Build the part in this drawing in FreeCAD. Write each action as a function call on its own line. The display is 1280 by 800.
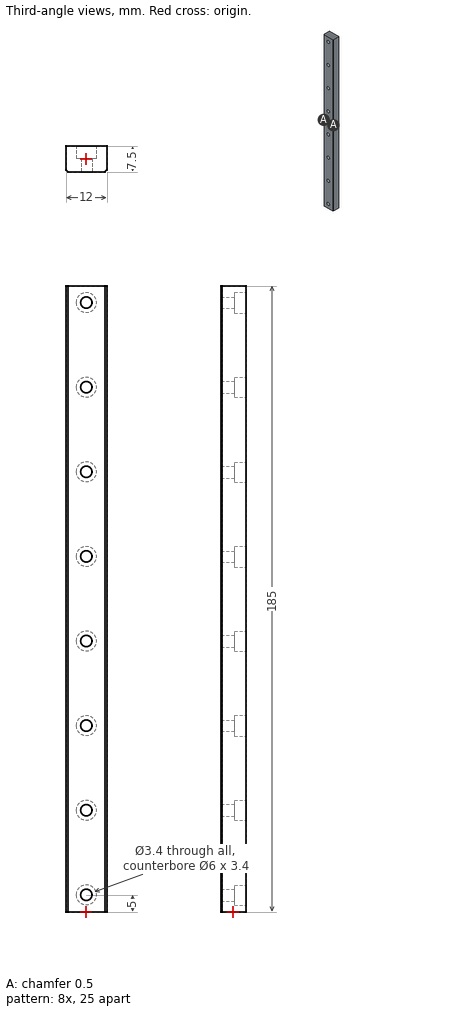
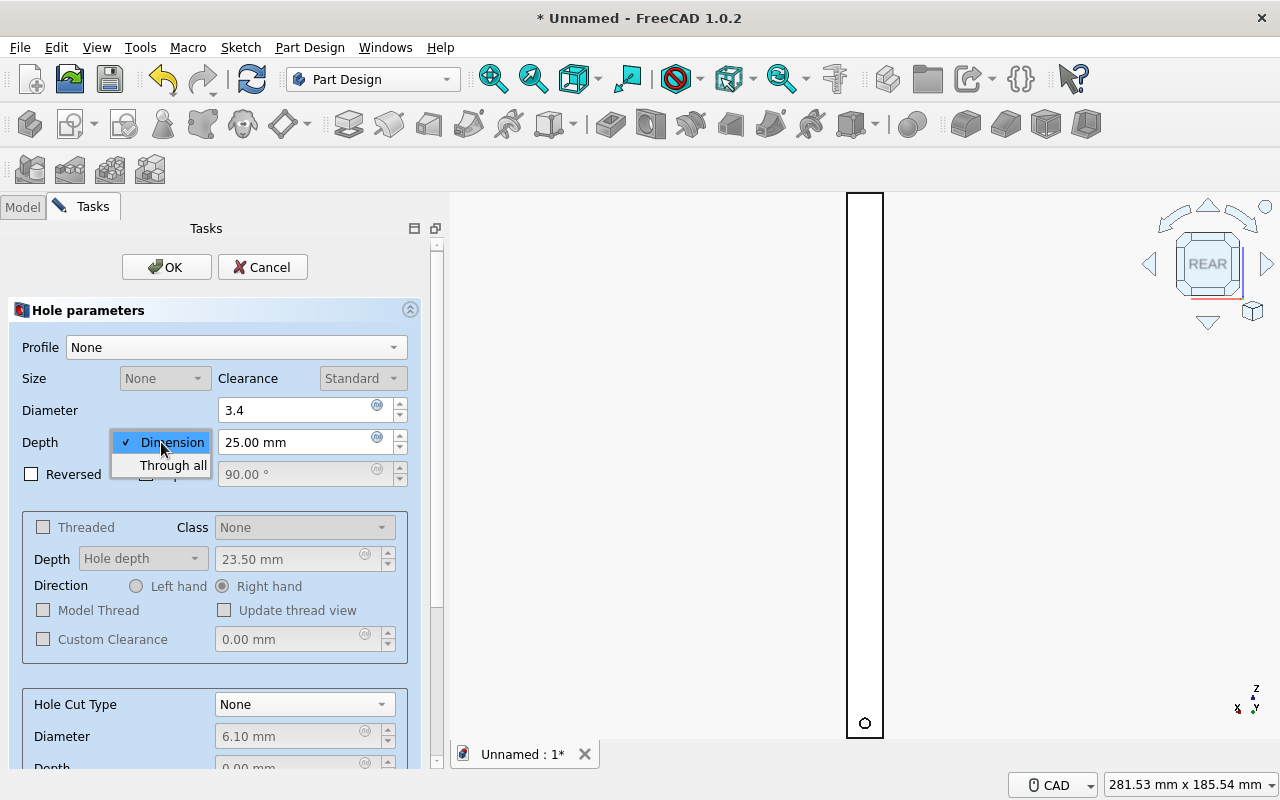
click(160, 466)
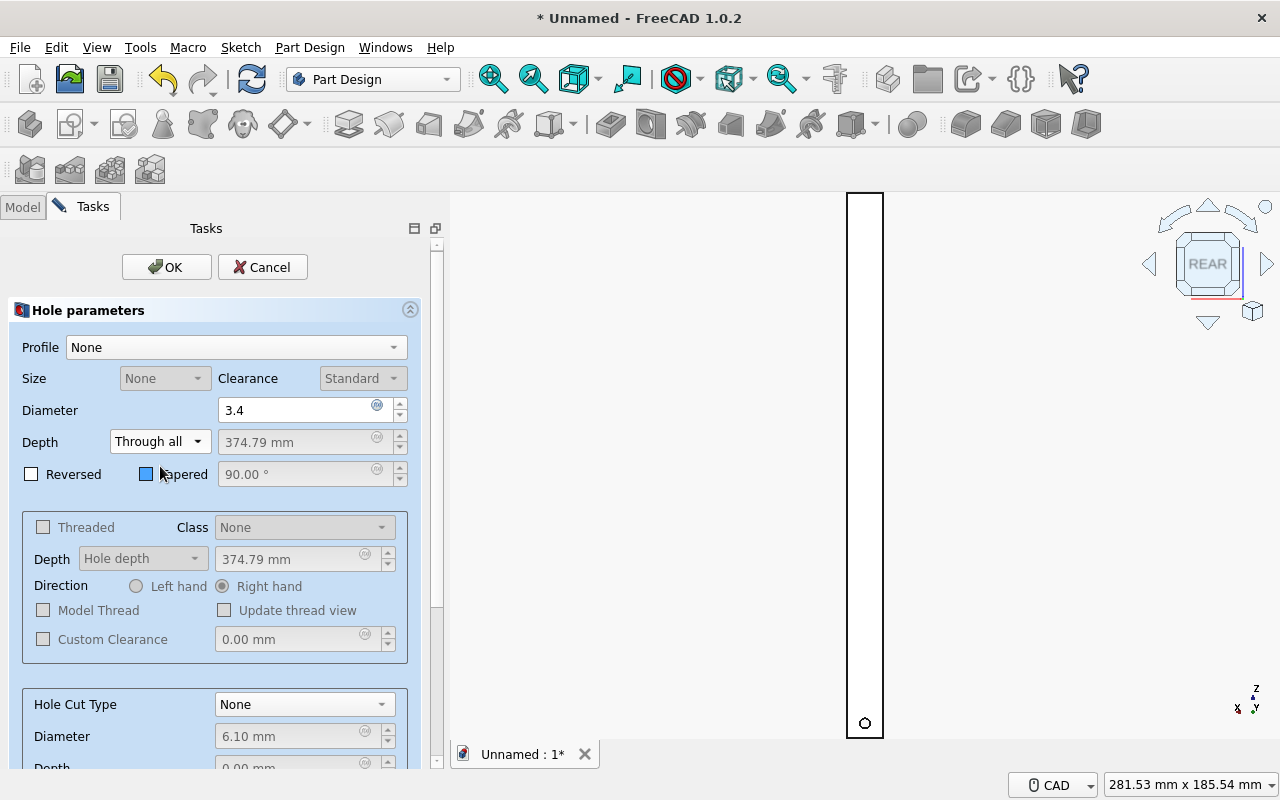
click(306, 704)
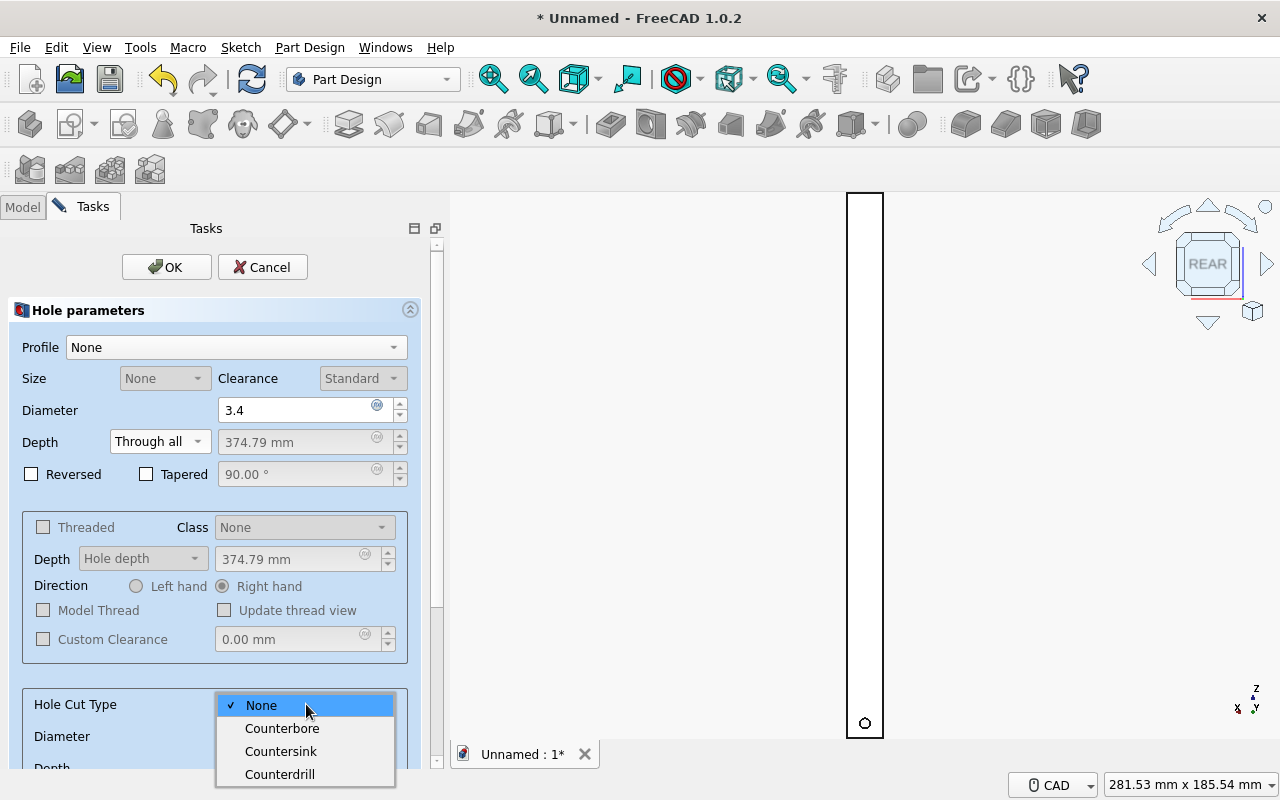
click(304, 728)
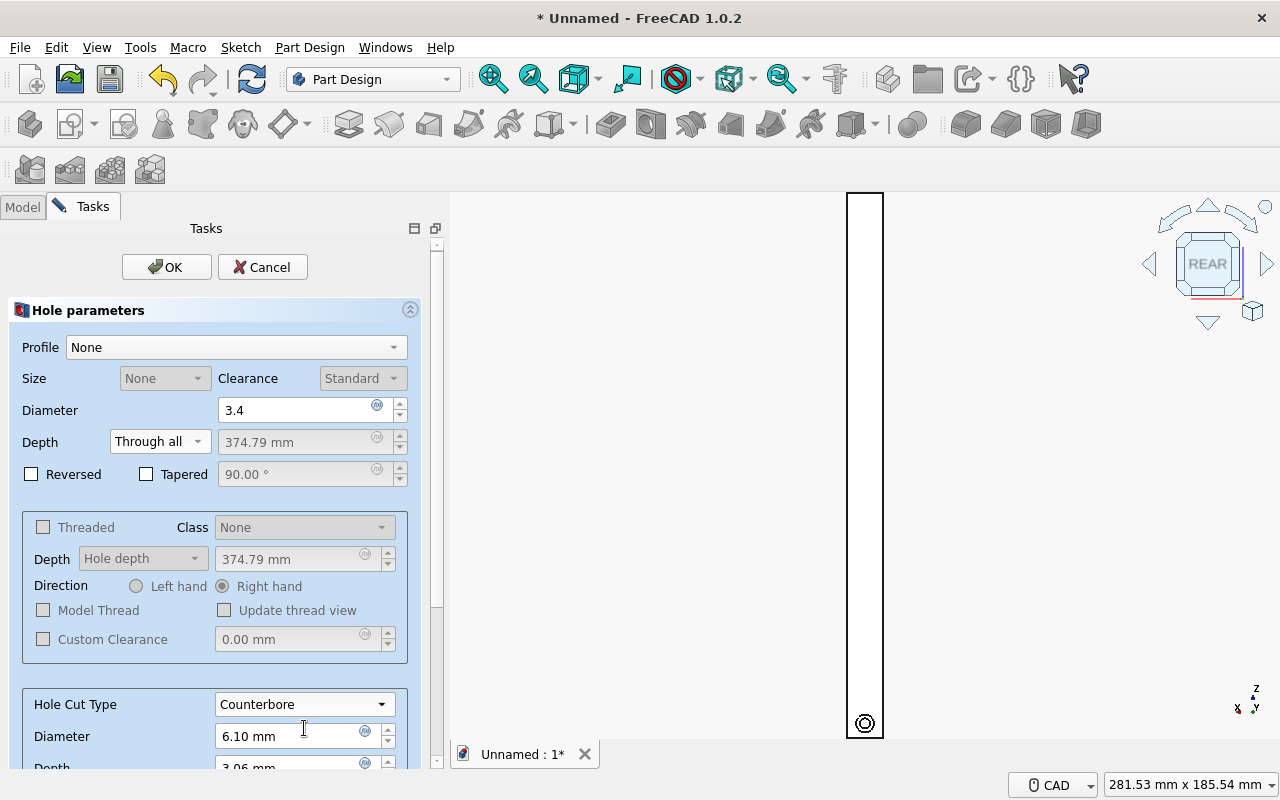
triple_click(298, 736)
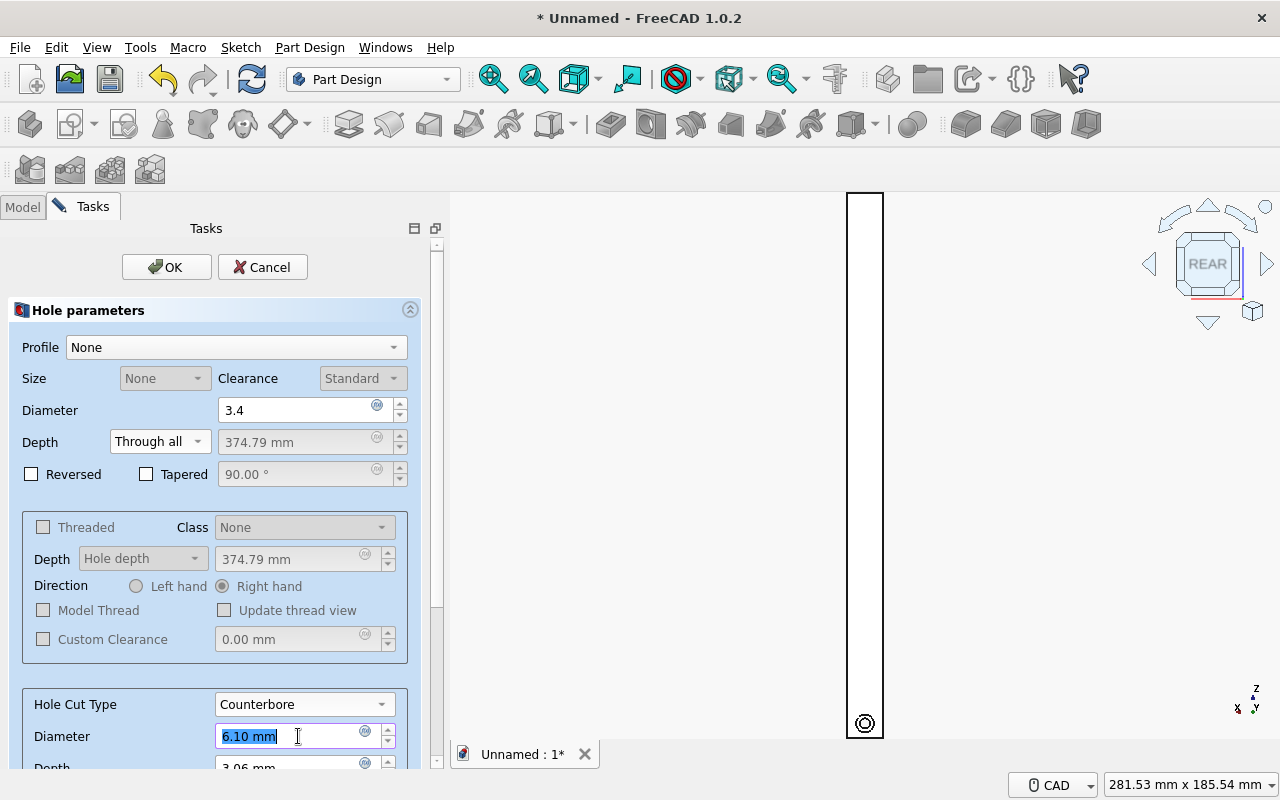
text(6)
key(Tab)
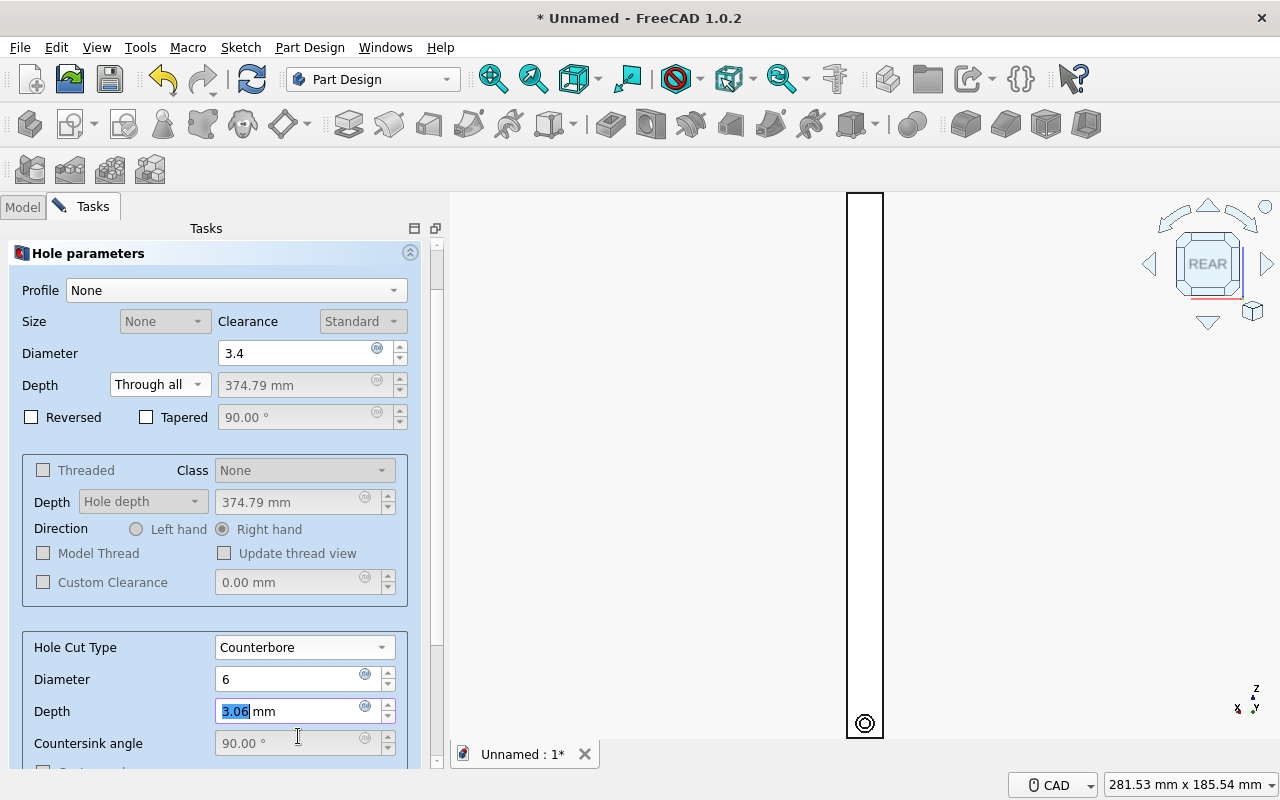
text(3.4)
key(Tab)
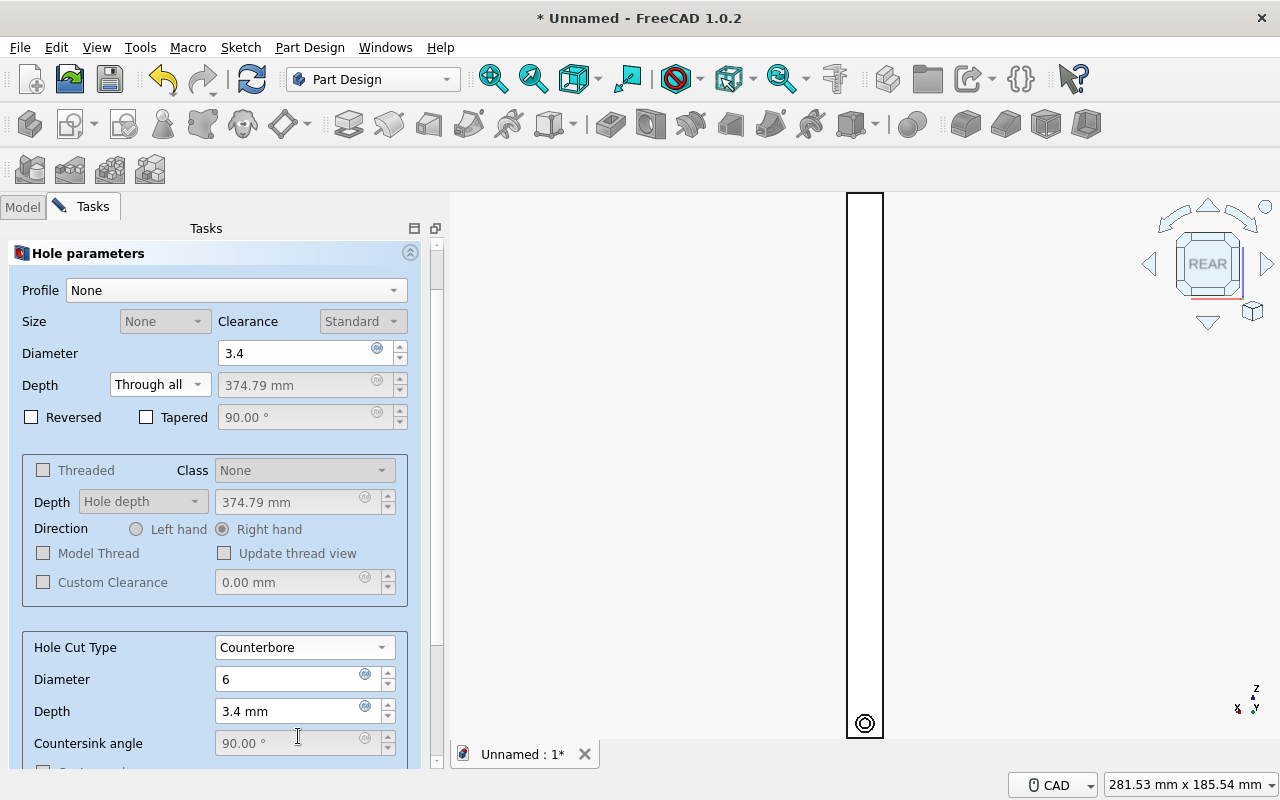
scroll(437, 503, up, 2)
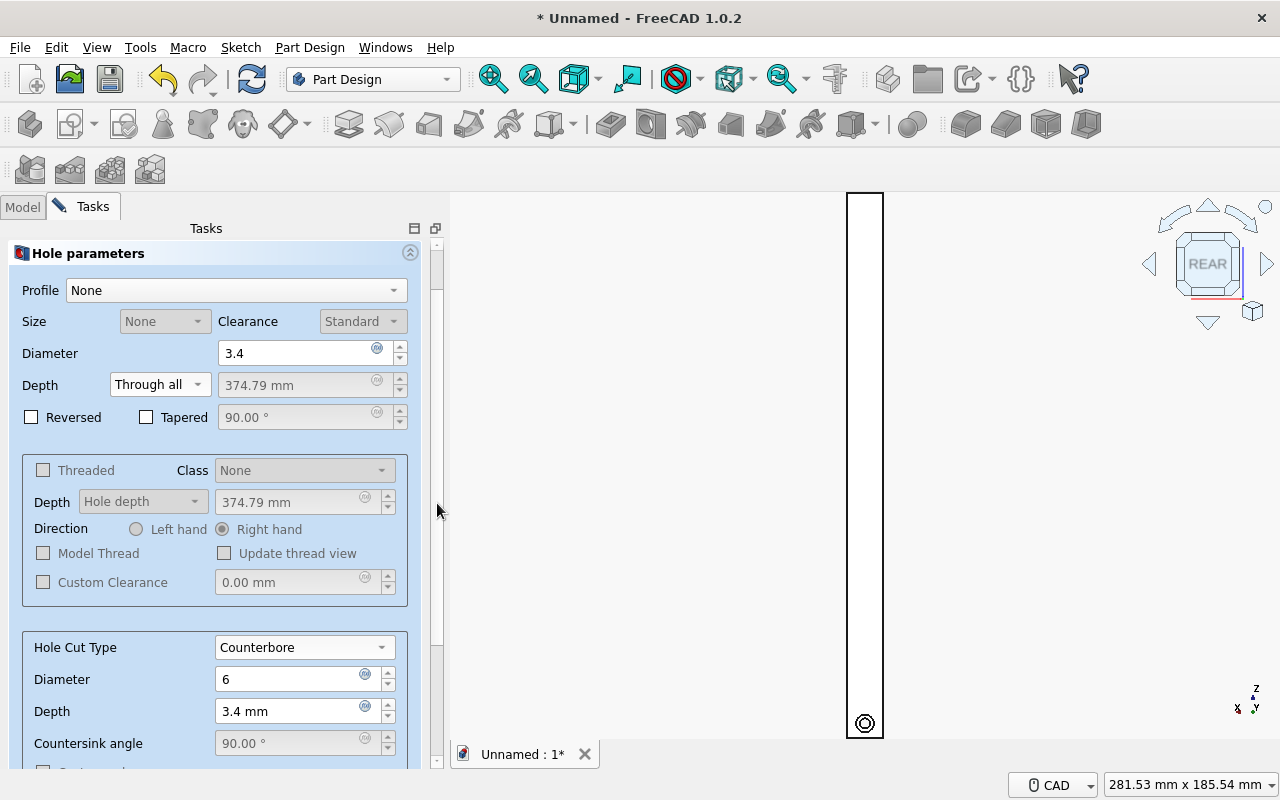
click(167, 267)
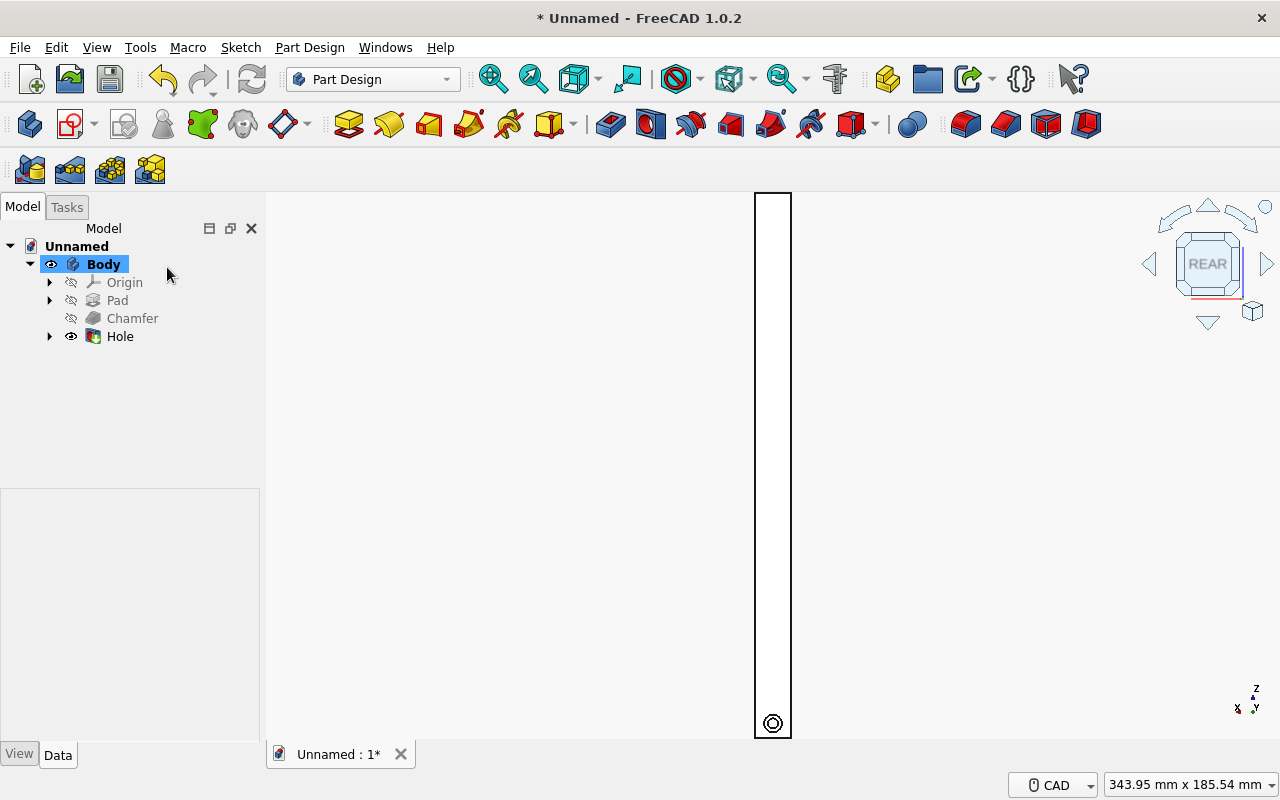
click(116, 336)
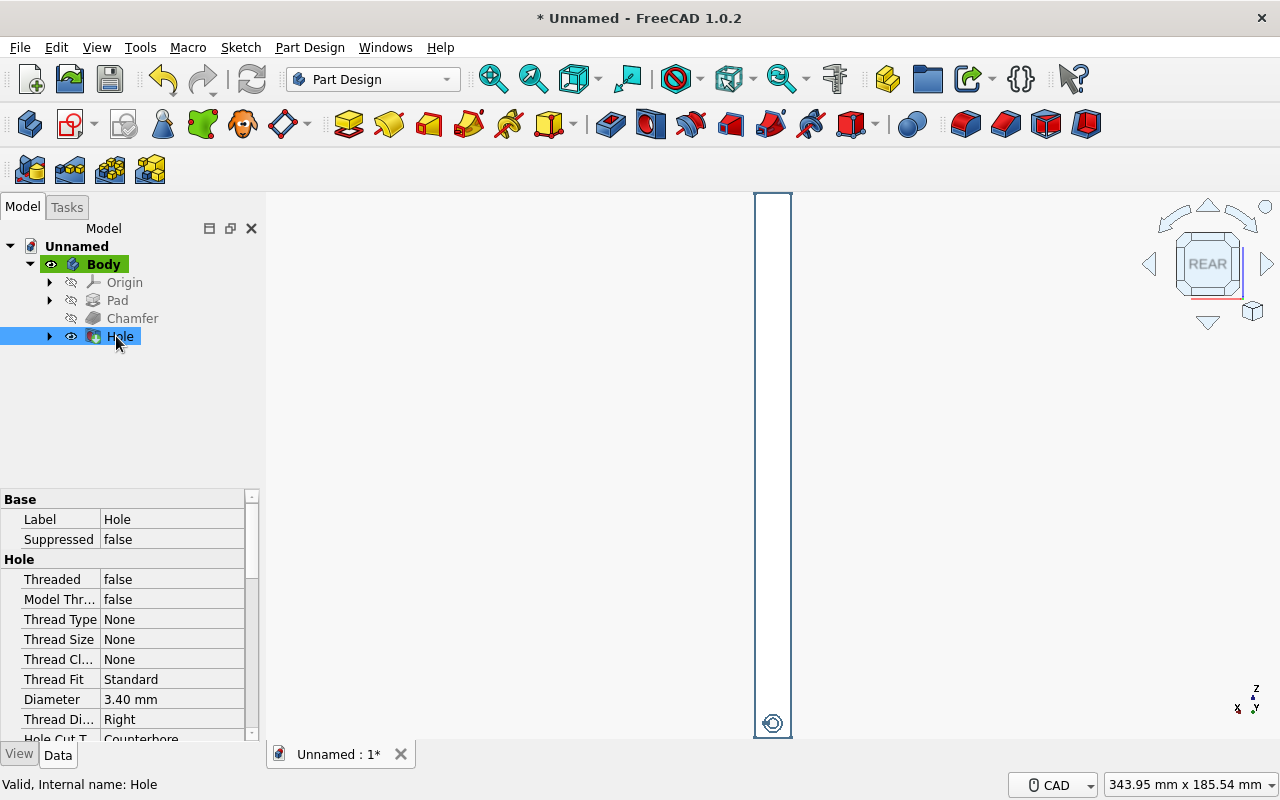
click(70, 170)